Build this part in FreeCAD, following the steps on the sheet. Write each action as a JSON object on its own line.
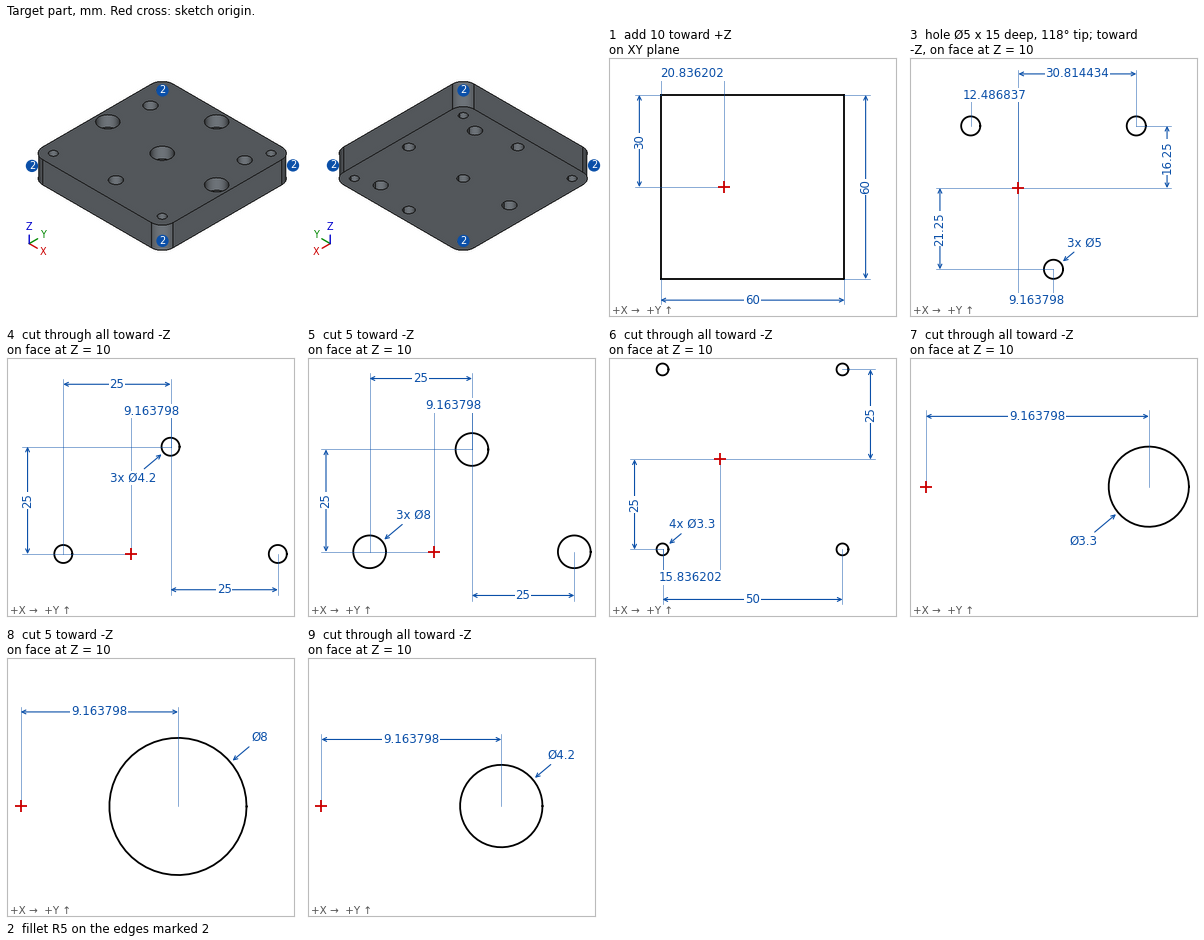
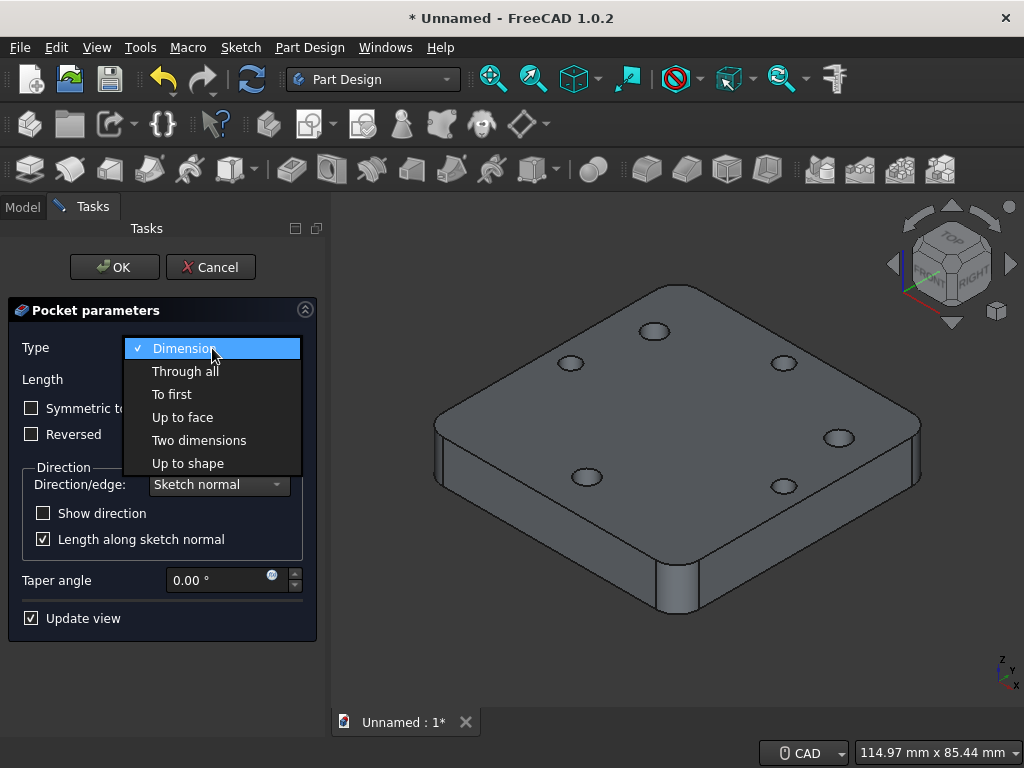
{"action": "left_click", "coordinate": [212, 372]}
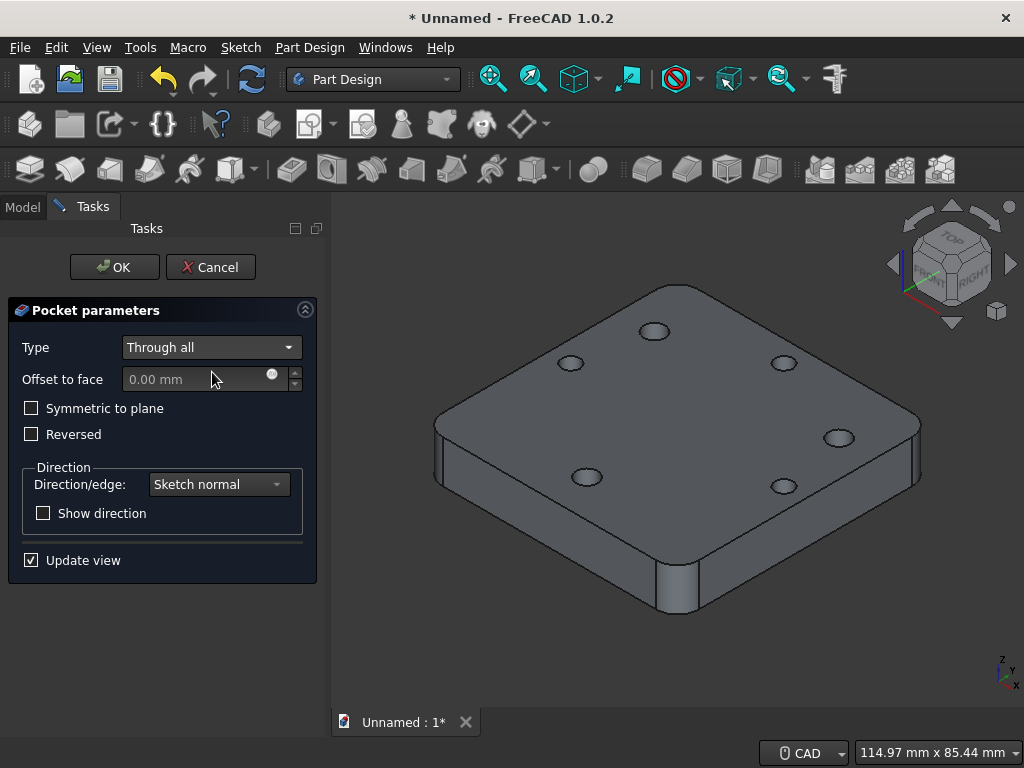
{"action": "left_click", "coordinate": [115, 267]}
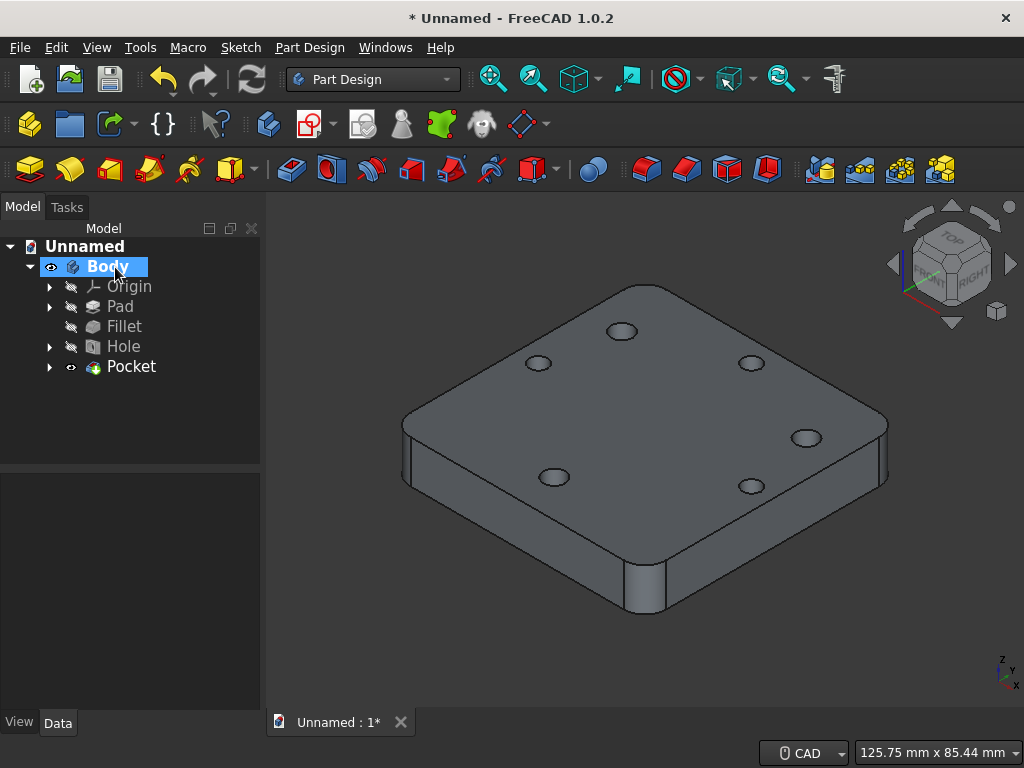
{"action": "left_click", "coordinate": [645, 424]}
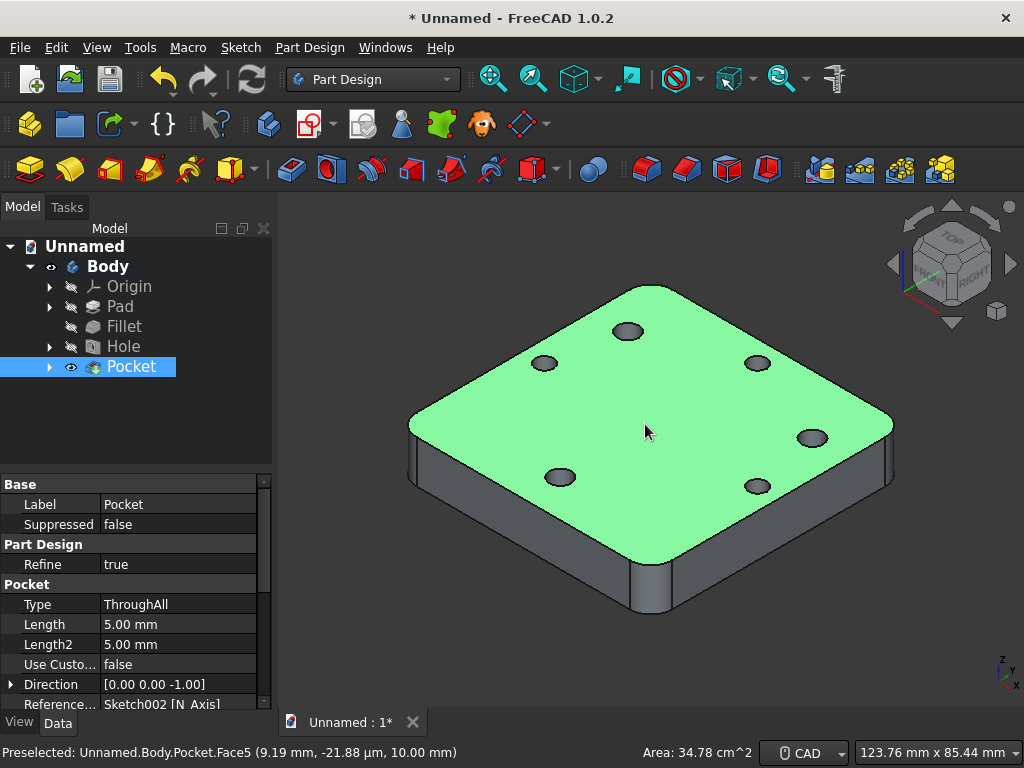
{"action": "left_click", "coordinate": [310, 124]}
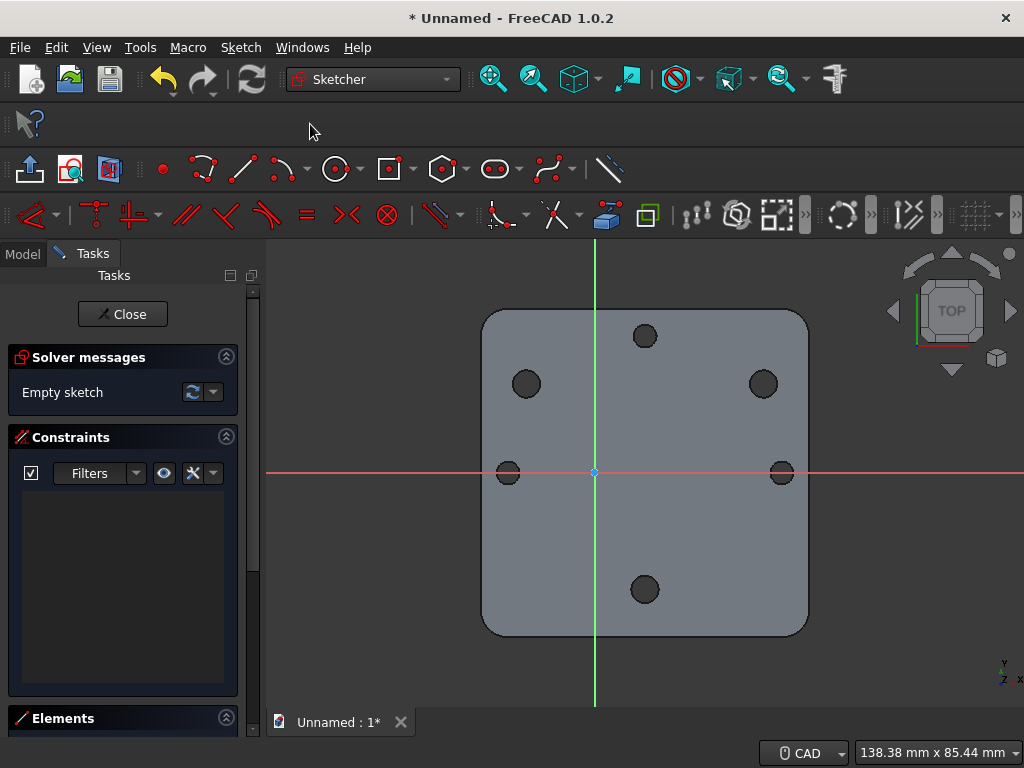
{"action": "left_click", "coordinate": [336, 170]}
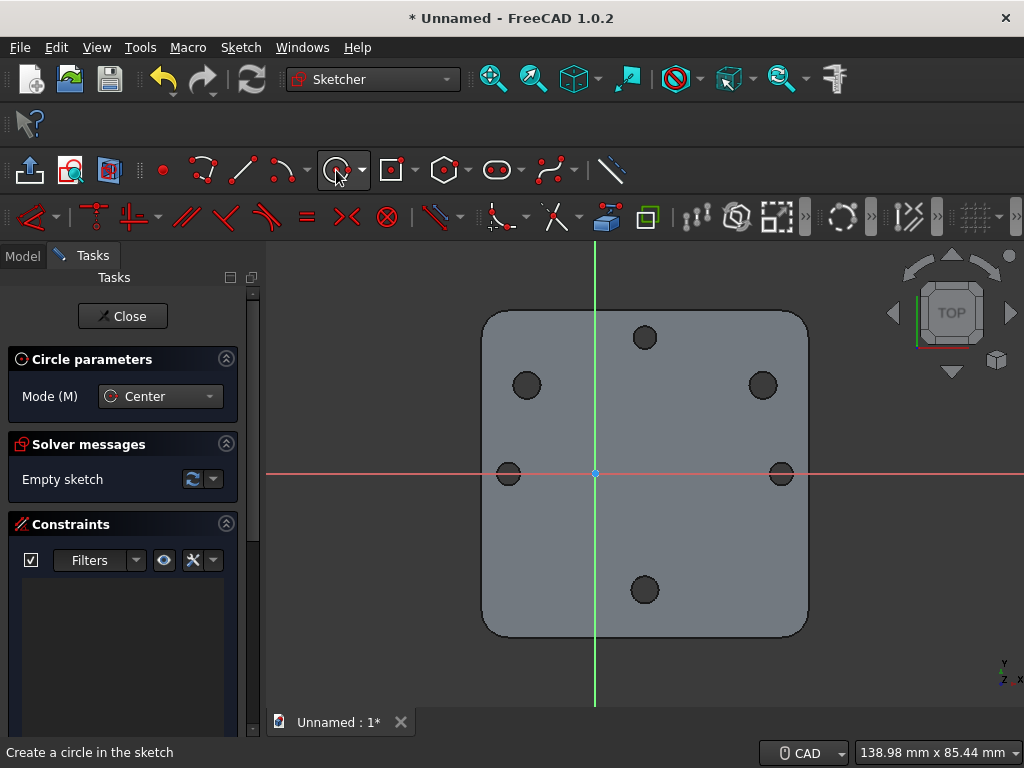
{"action": "left_click", "coordinate": [509, 474]}
{"action": "mouse_move", "coordinate": [524, 459]}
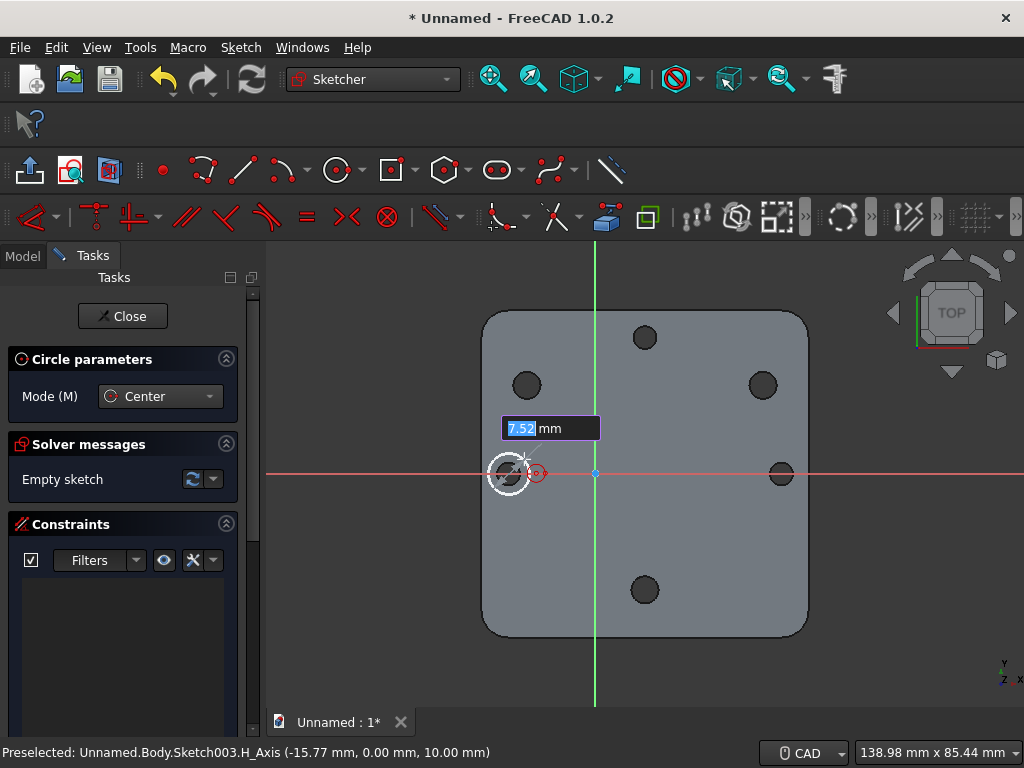
{"action": "type", "text": "8"}
{"action": "key", "text": "Return"}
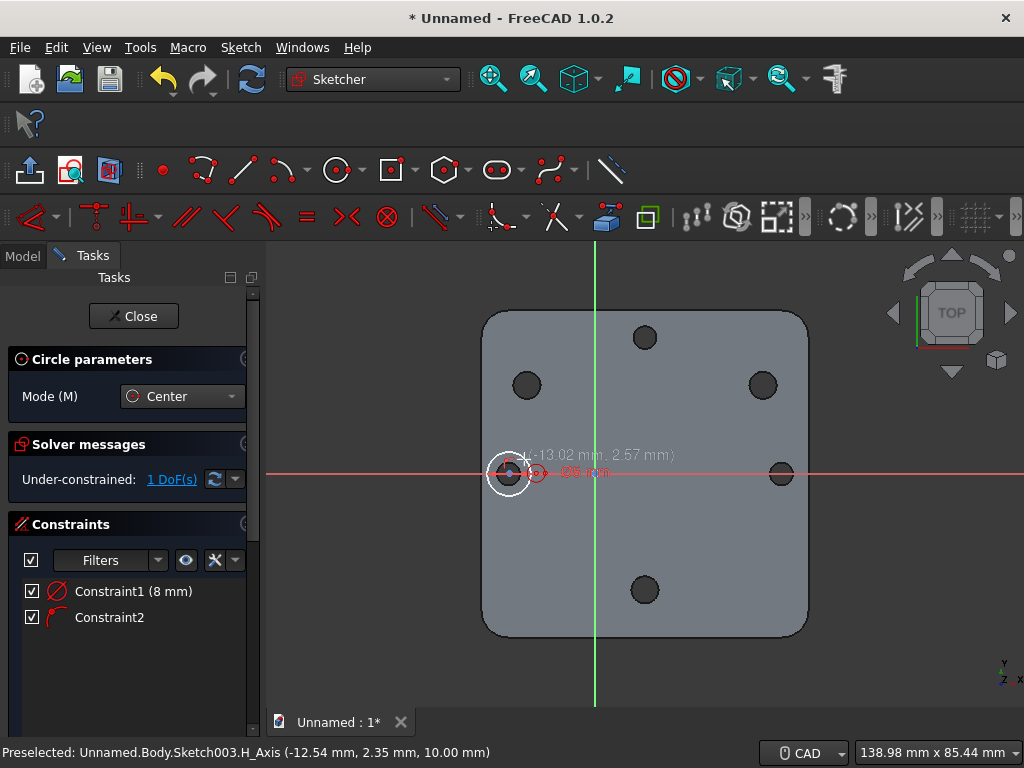
{"action": "left_click", "coordinate": [645, 338]}
{"action": "mouse_move", "coordinate": [660, 322]}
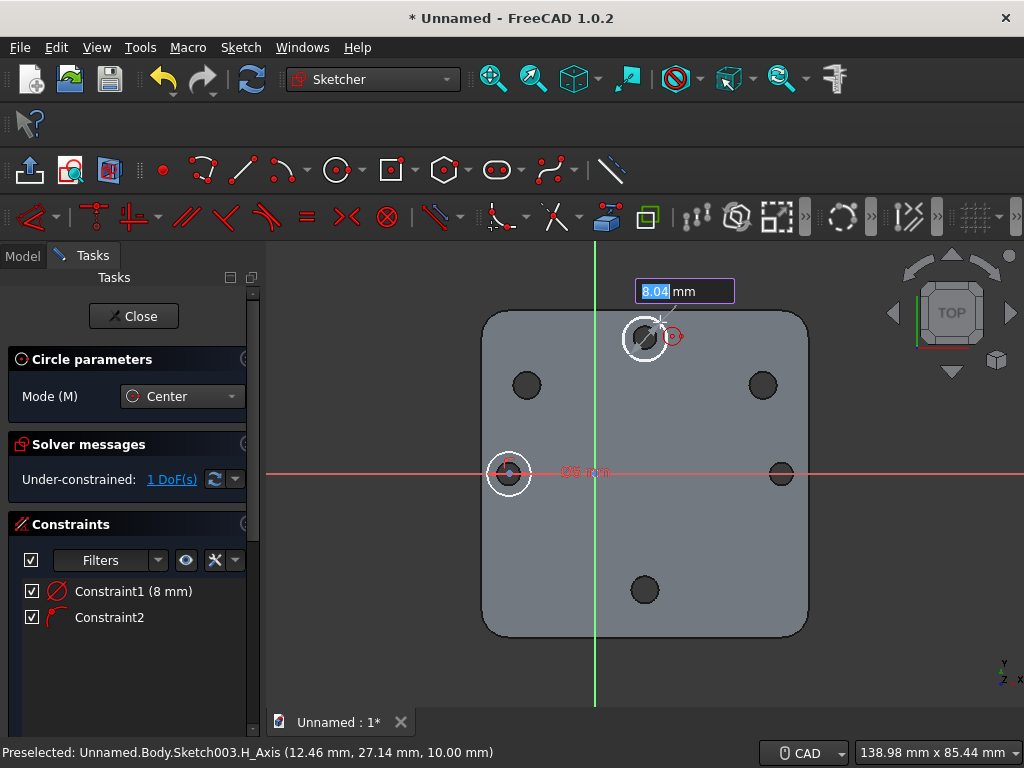
{"action": "type", "text": "8"}
{"action": "key", "text": "Return"}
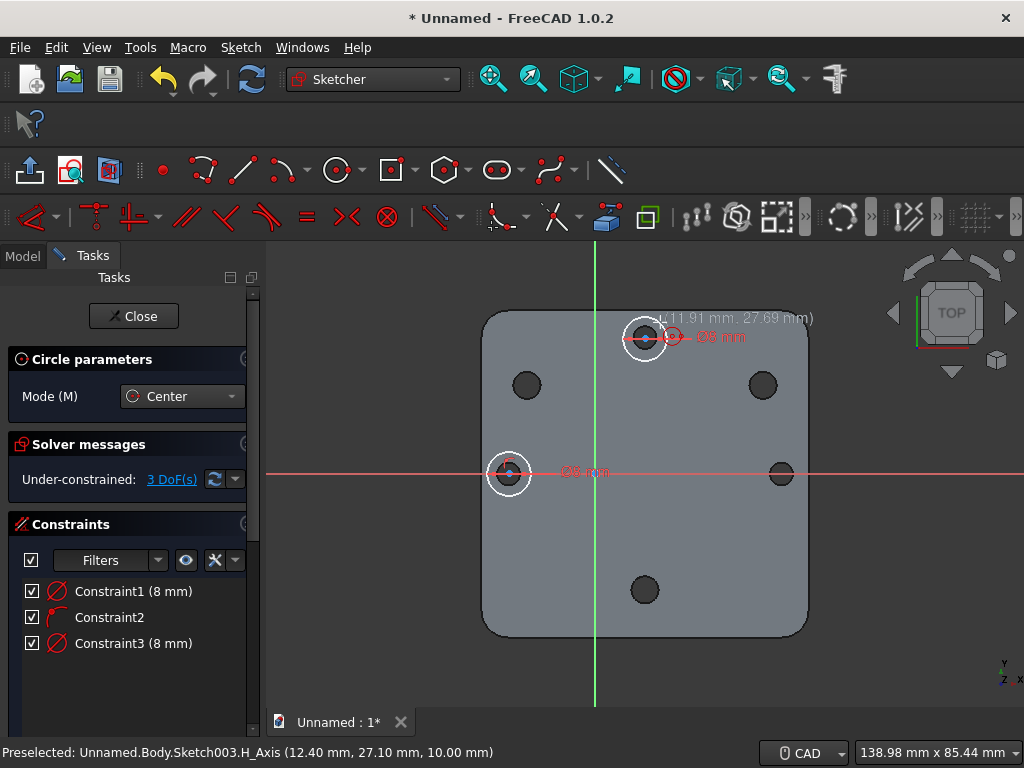
{"action": "left_click", "coordinate": [781, 474]}
{"action": "mouse_move", "coordinate": [797, 459]}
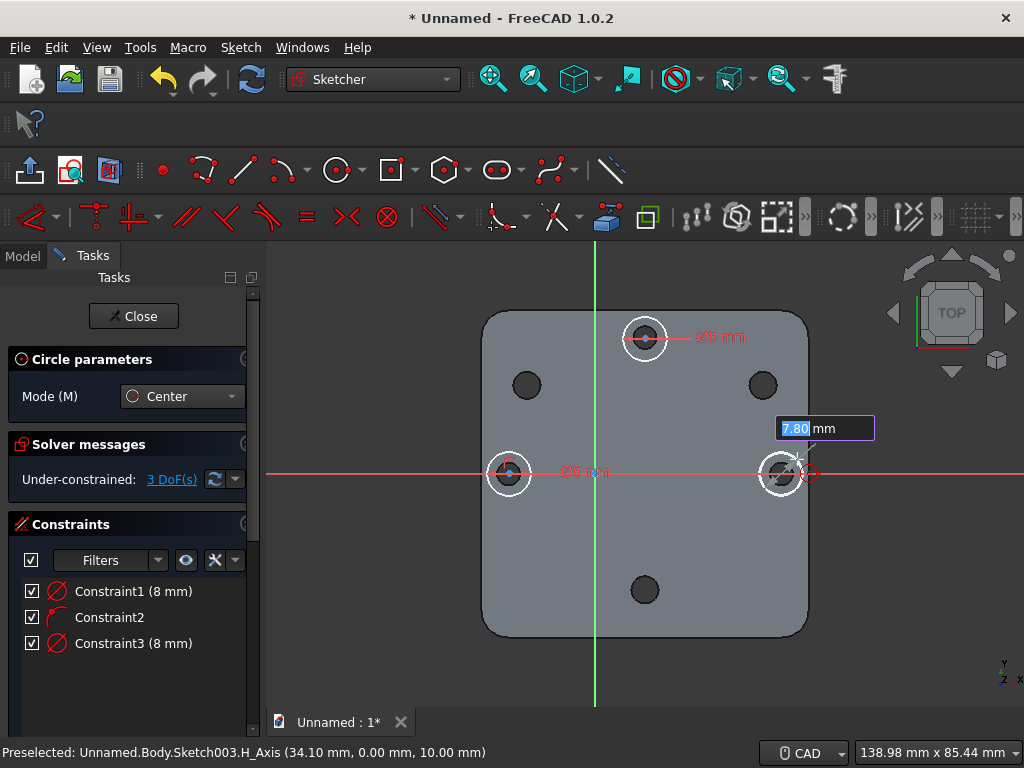
{"action": "type", "text": "8"}
{"action": "key", "text": "Return"}
{"action": "key", "text": "Escape"}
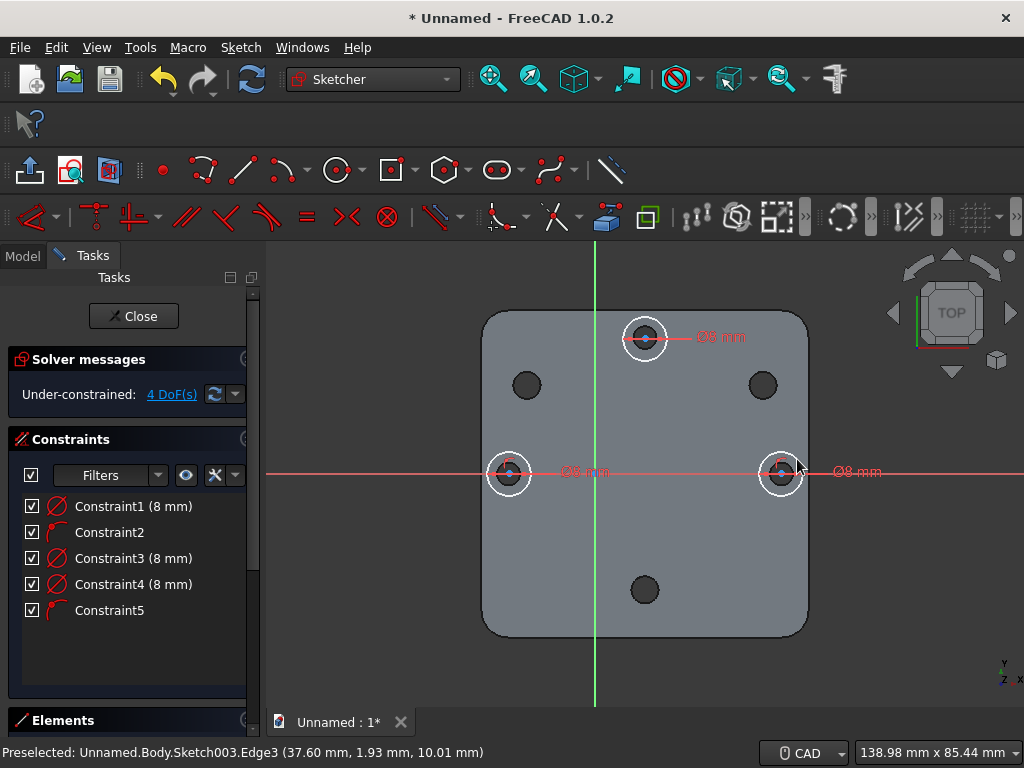
{"action": "left_click", "coordinate": [32, 218]}